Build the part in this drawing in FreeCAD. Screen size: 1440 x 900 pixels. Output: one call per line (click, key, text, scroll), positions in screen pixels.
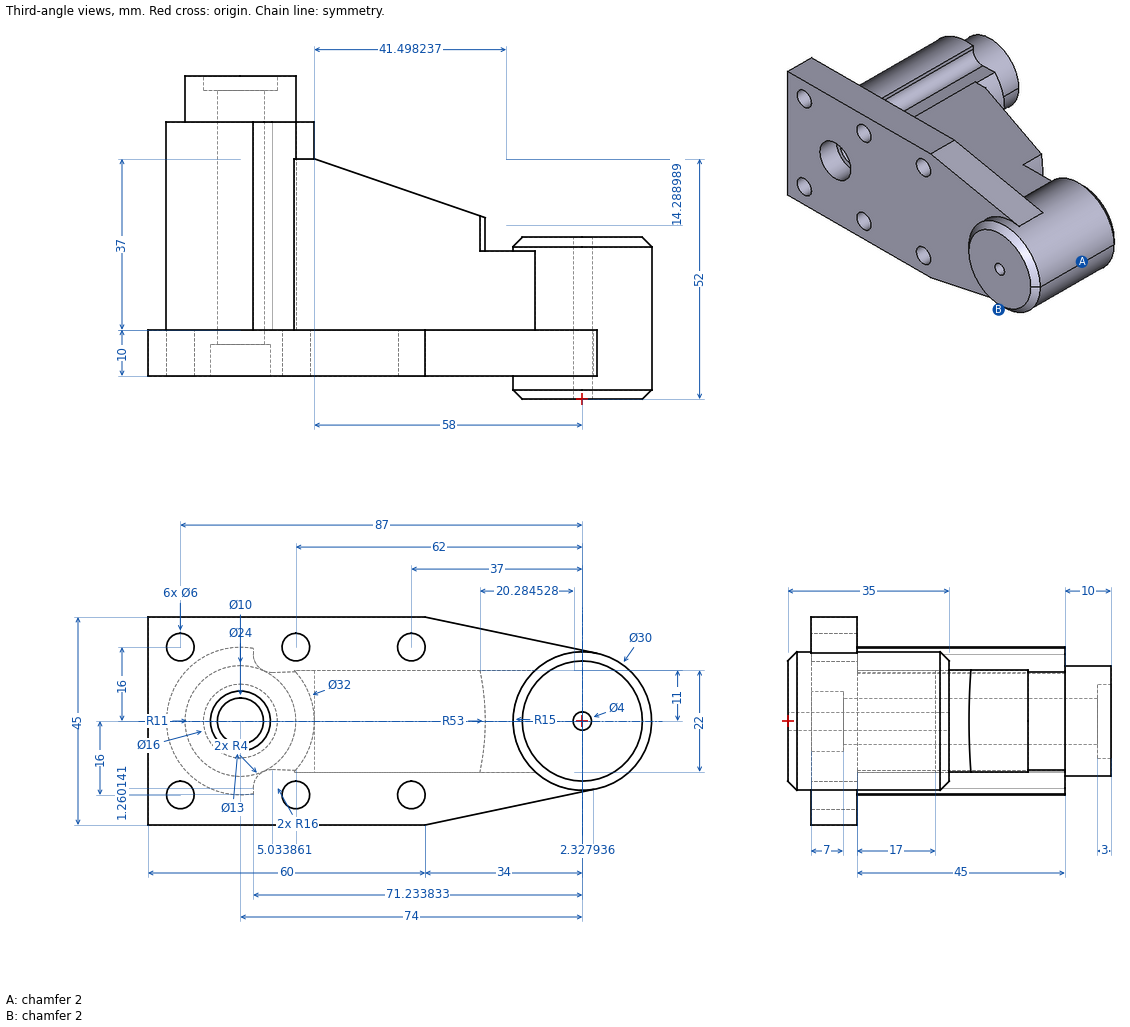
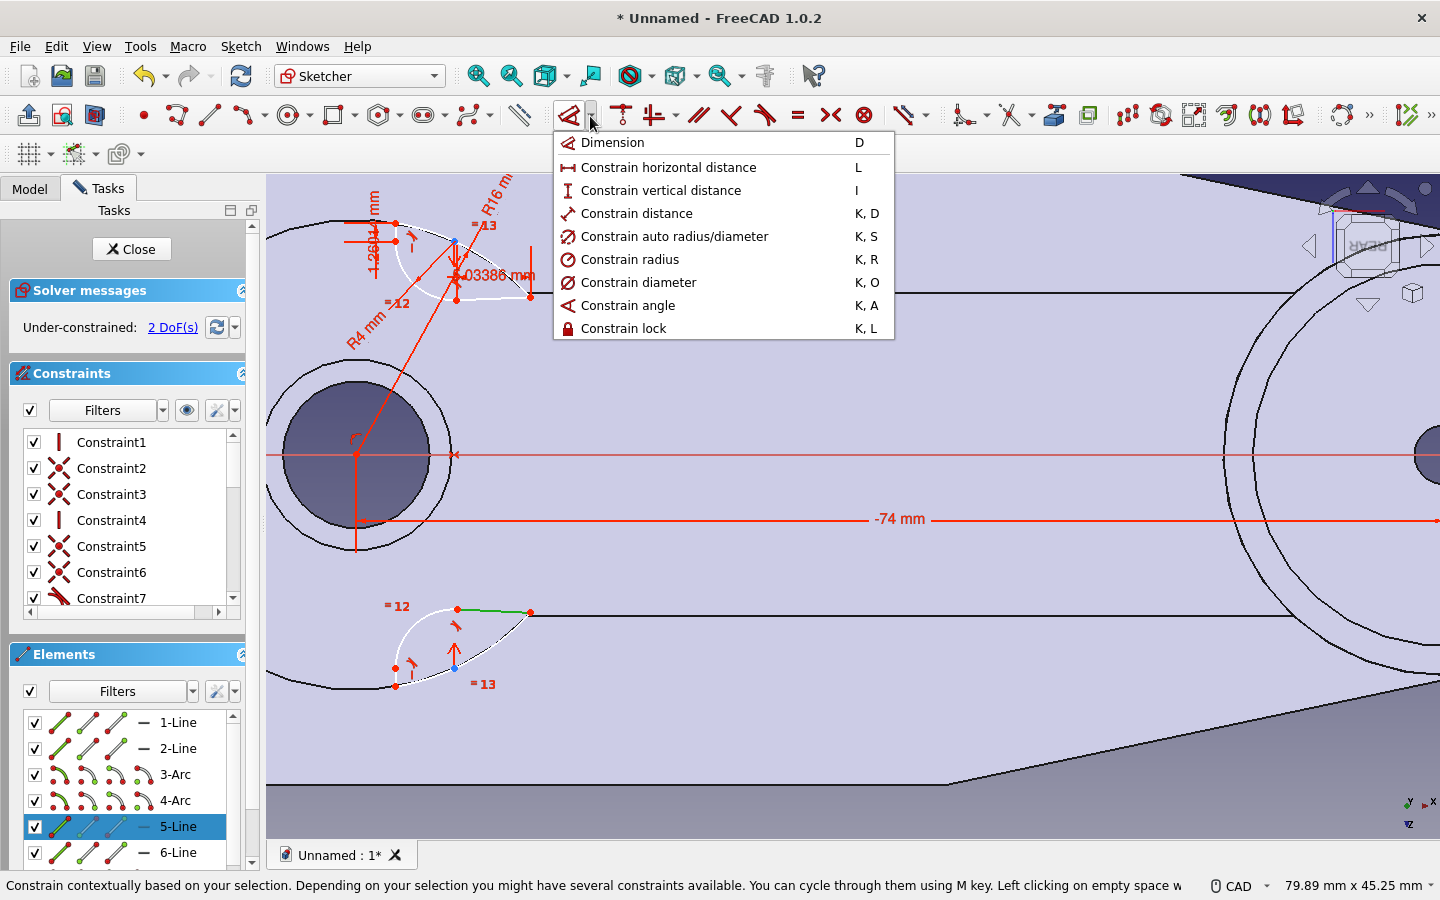
click(724, 168)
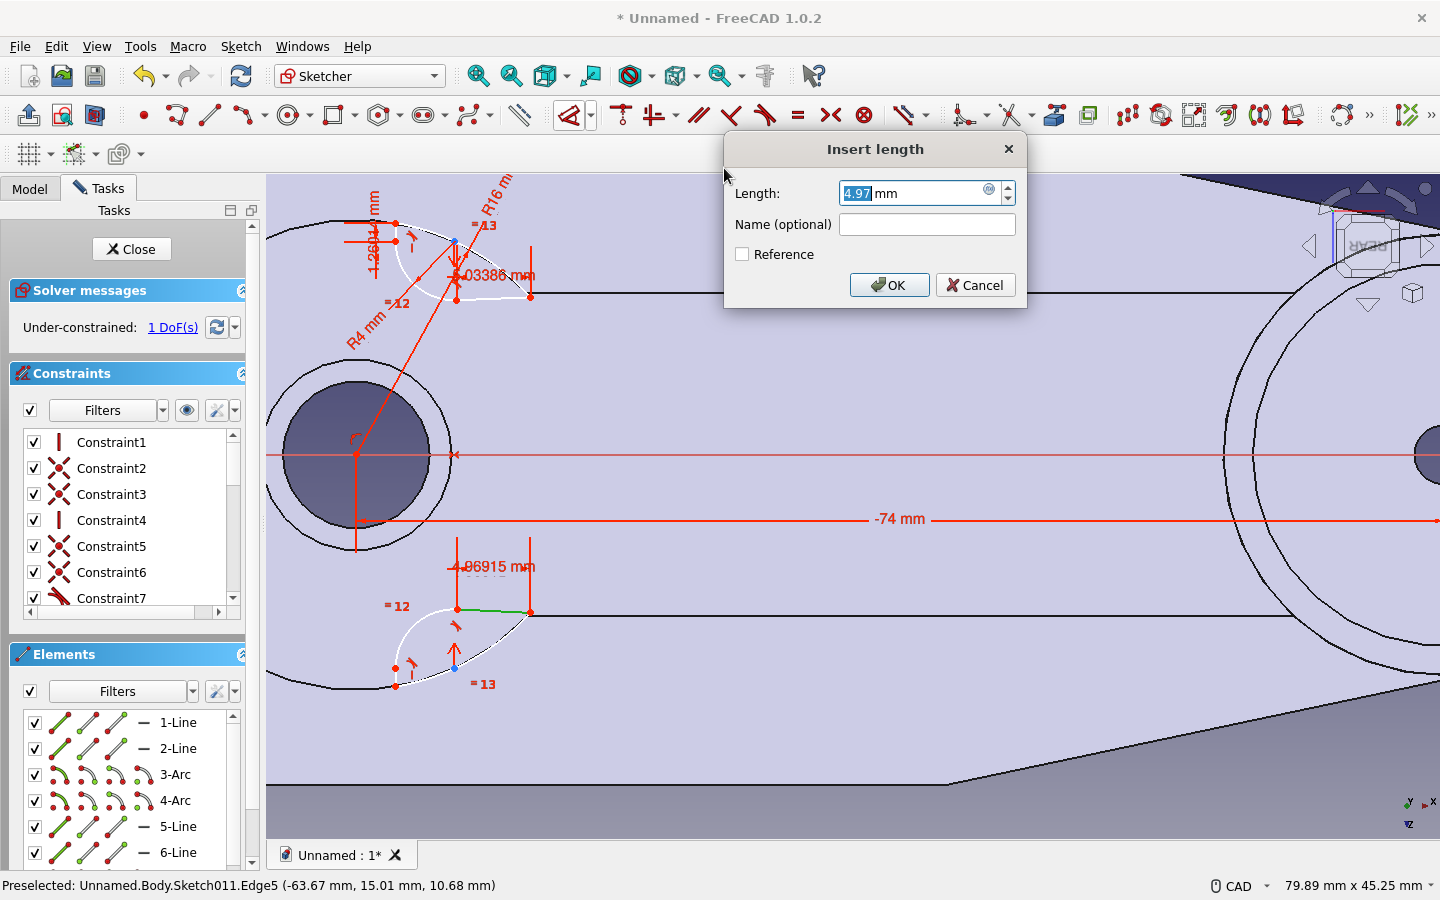
text(5.033861)
key(Return)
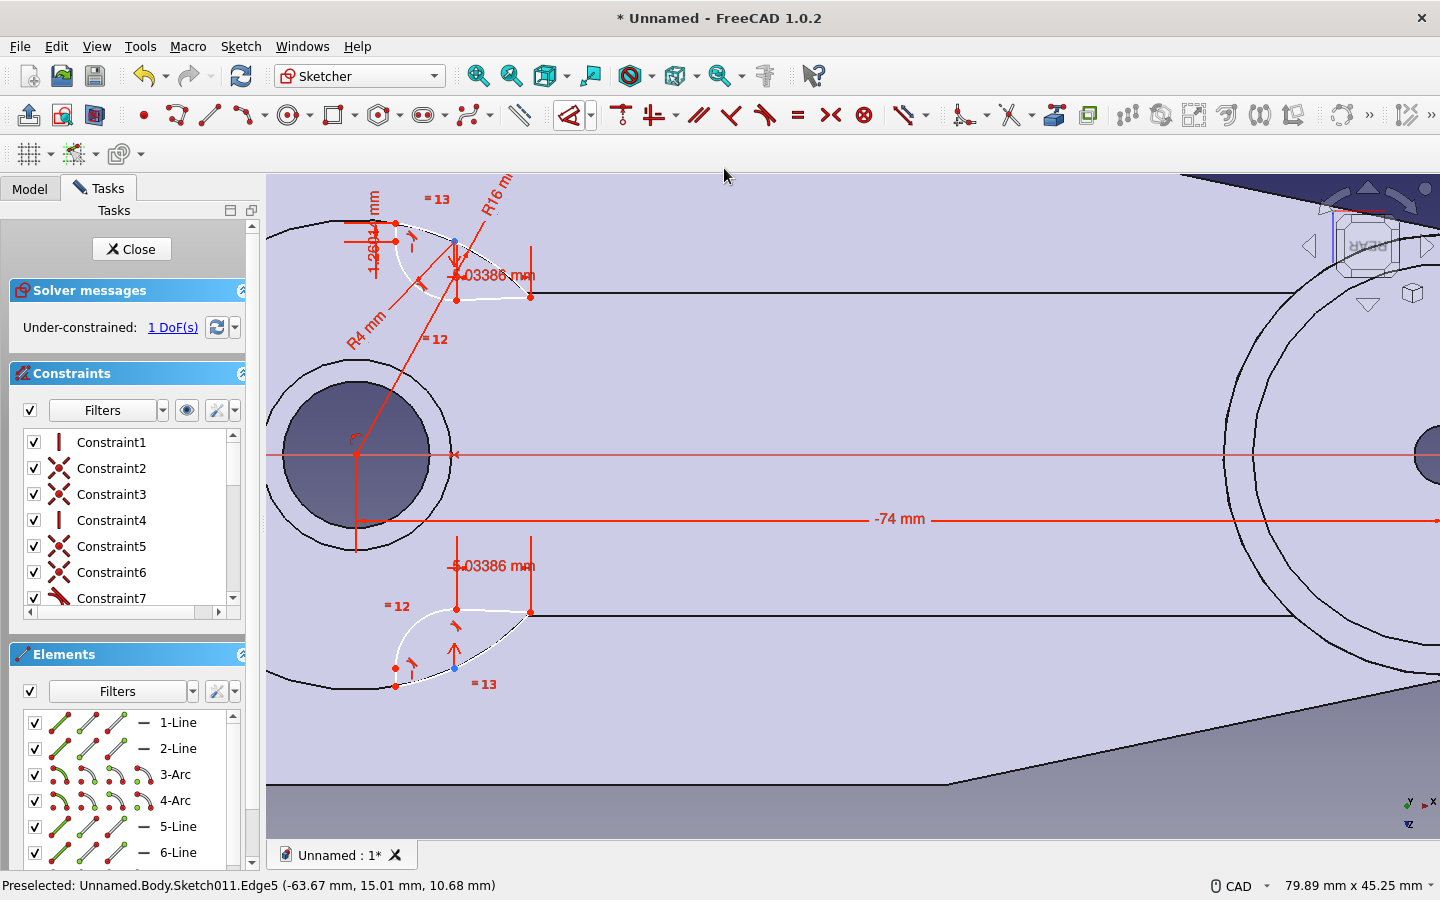
click(396, 223)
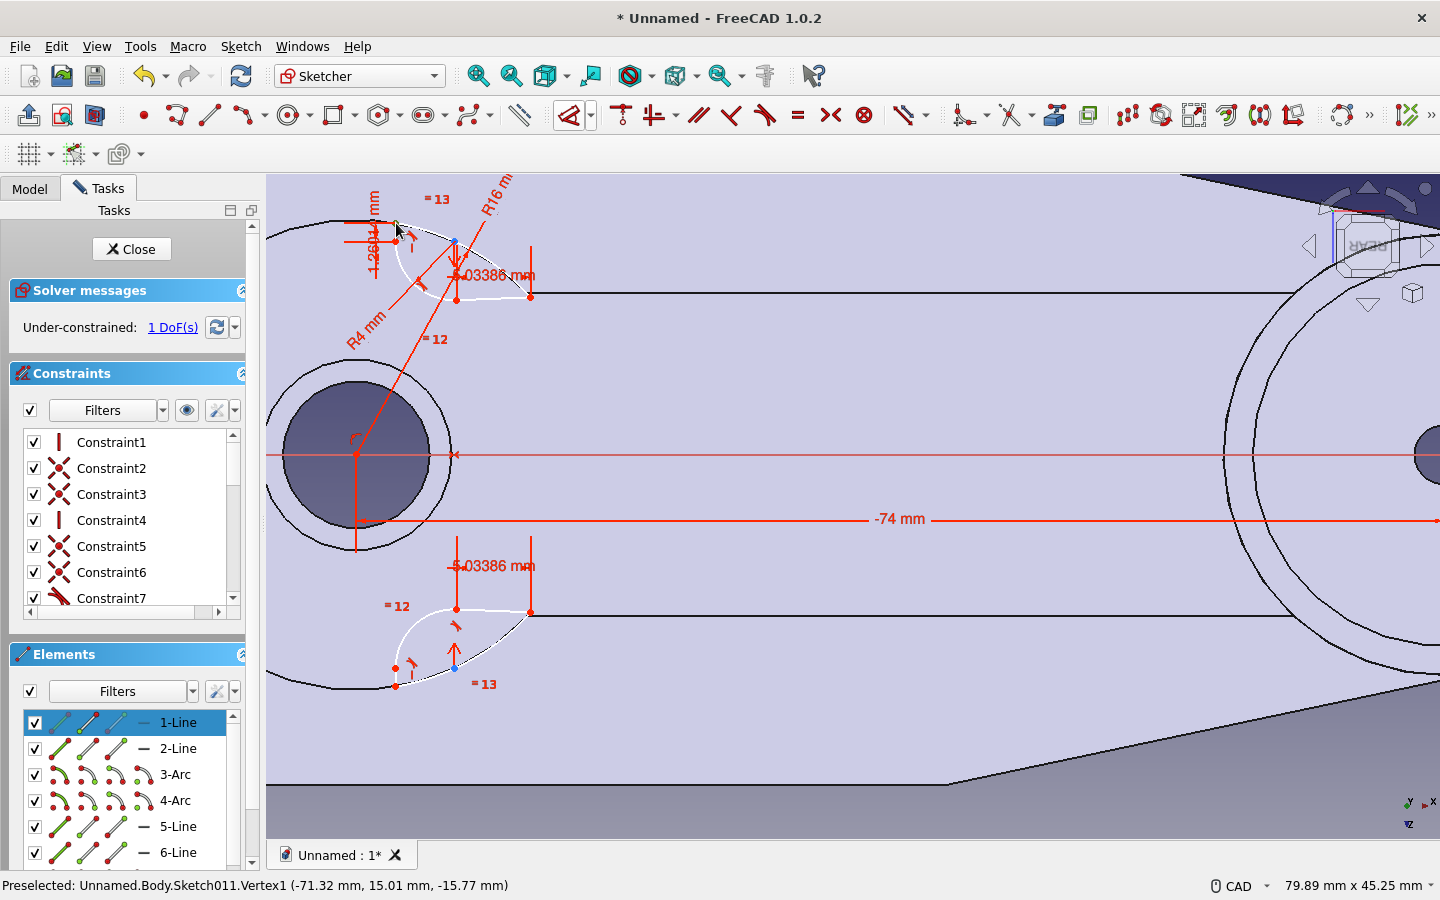
click(590, 116)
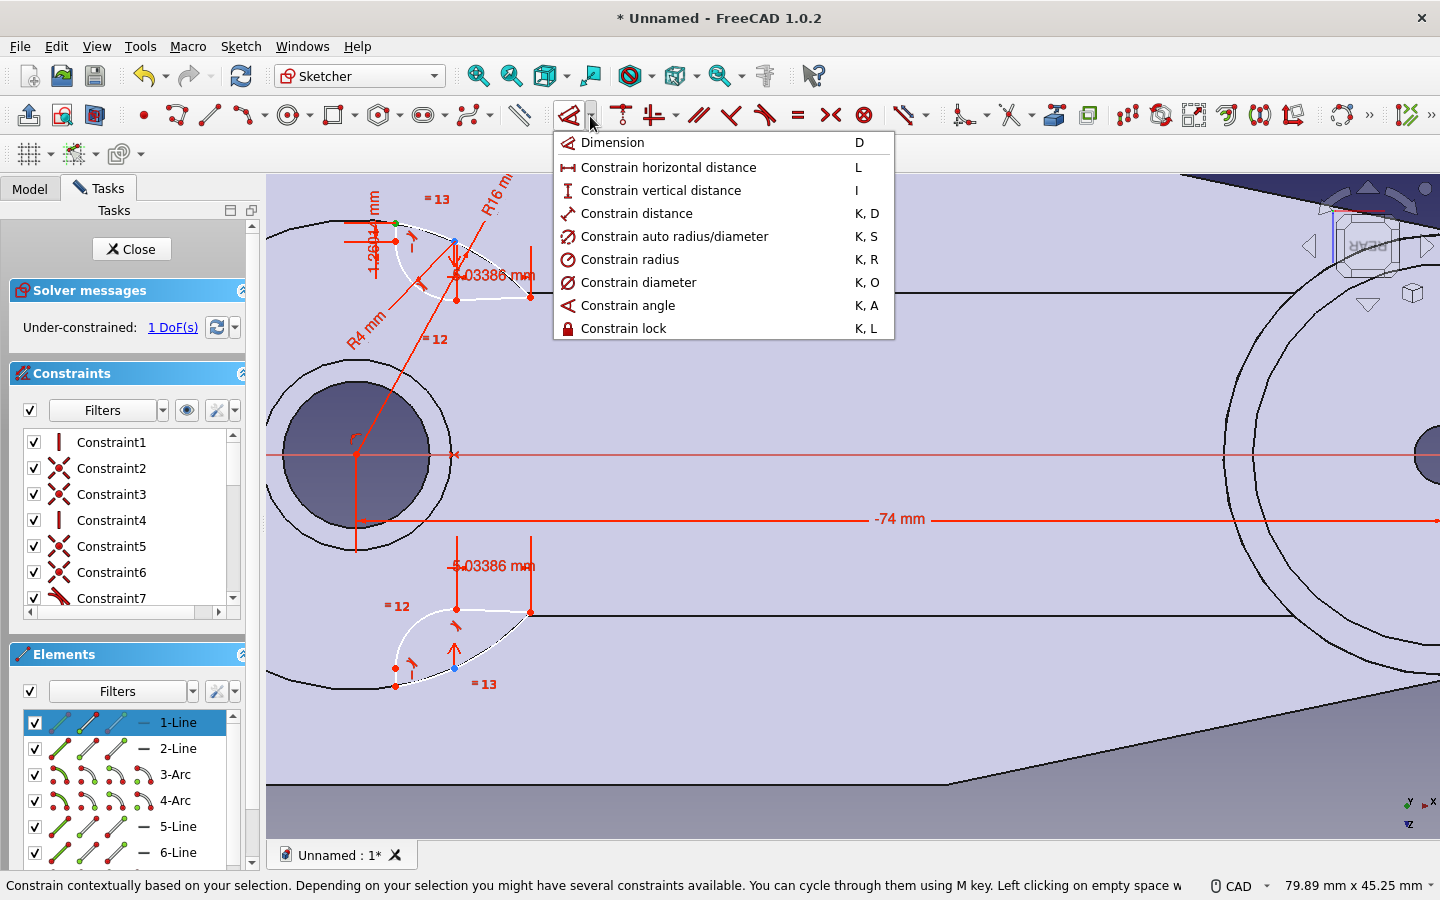
click(724, 168)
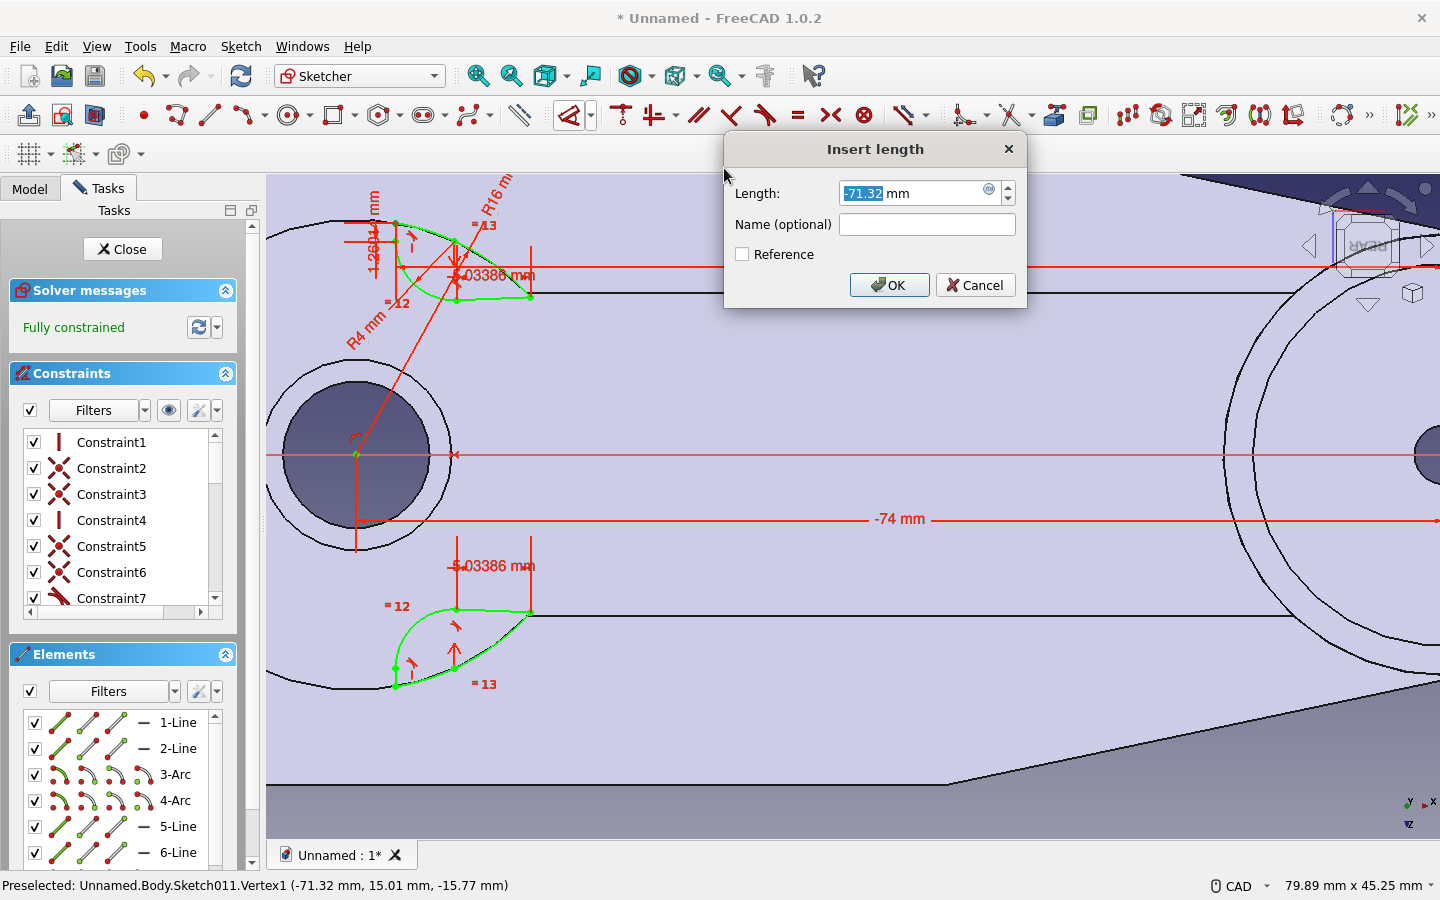
text(-71.233833)
key(Return)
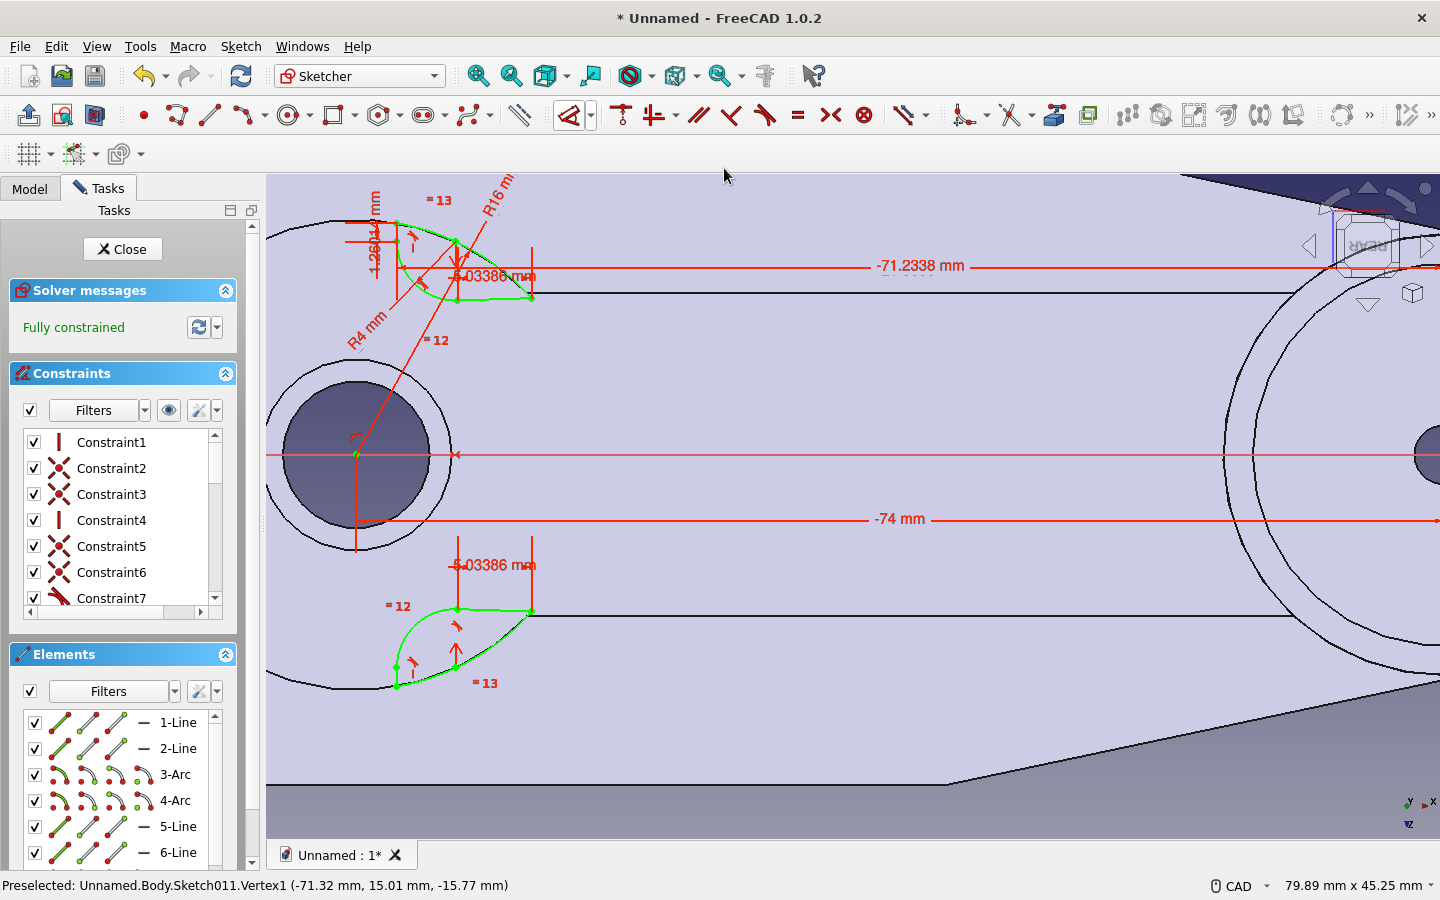
click(123, 249)